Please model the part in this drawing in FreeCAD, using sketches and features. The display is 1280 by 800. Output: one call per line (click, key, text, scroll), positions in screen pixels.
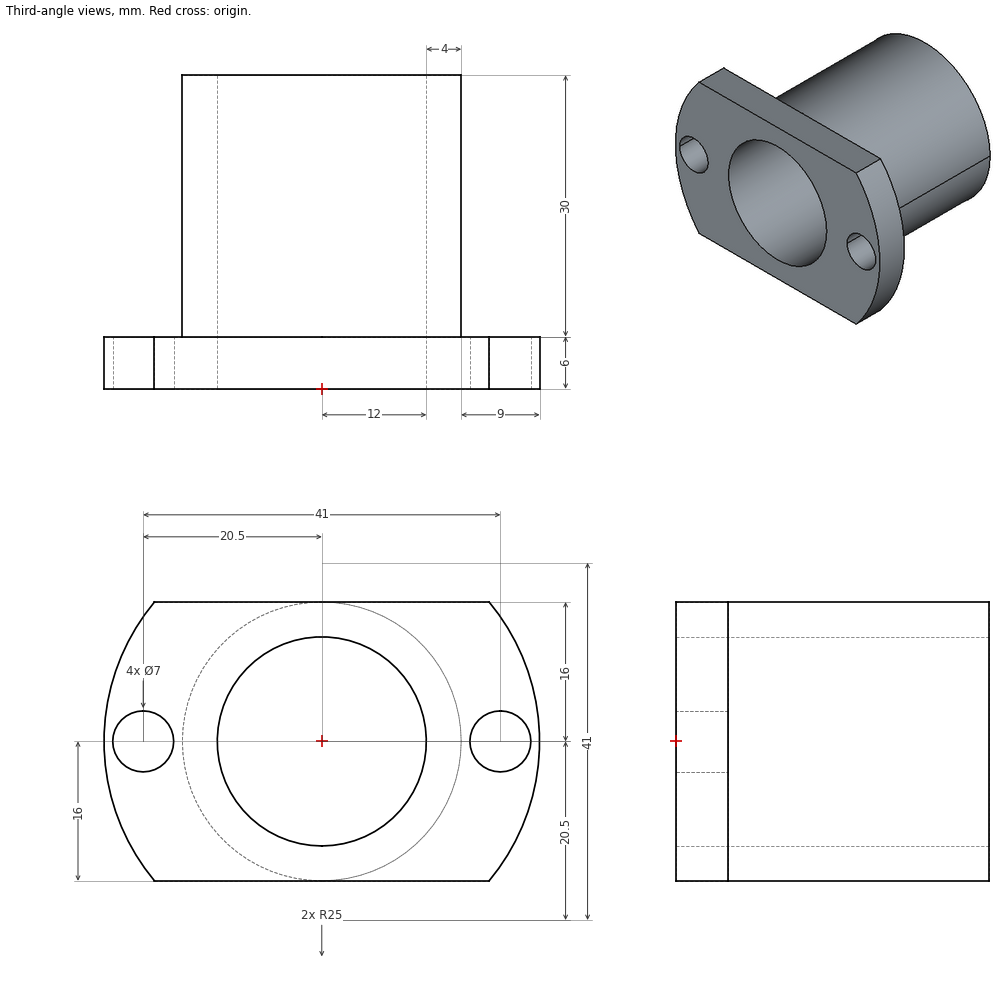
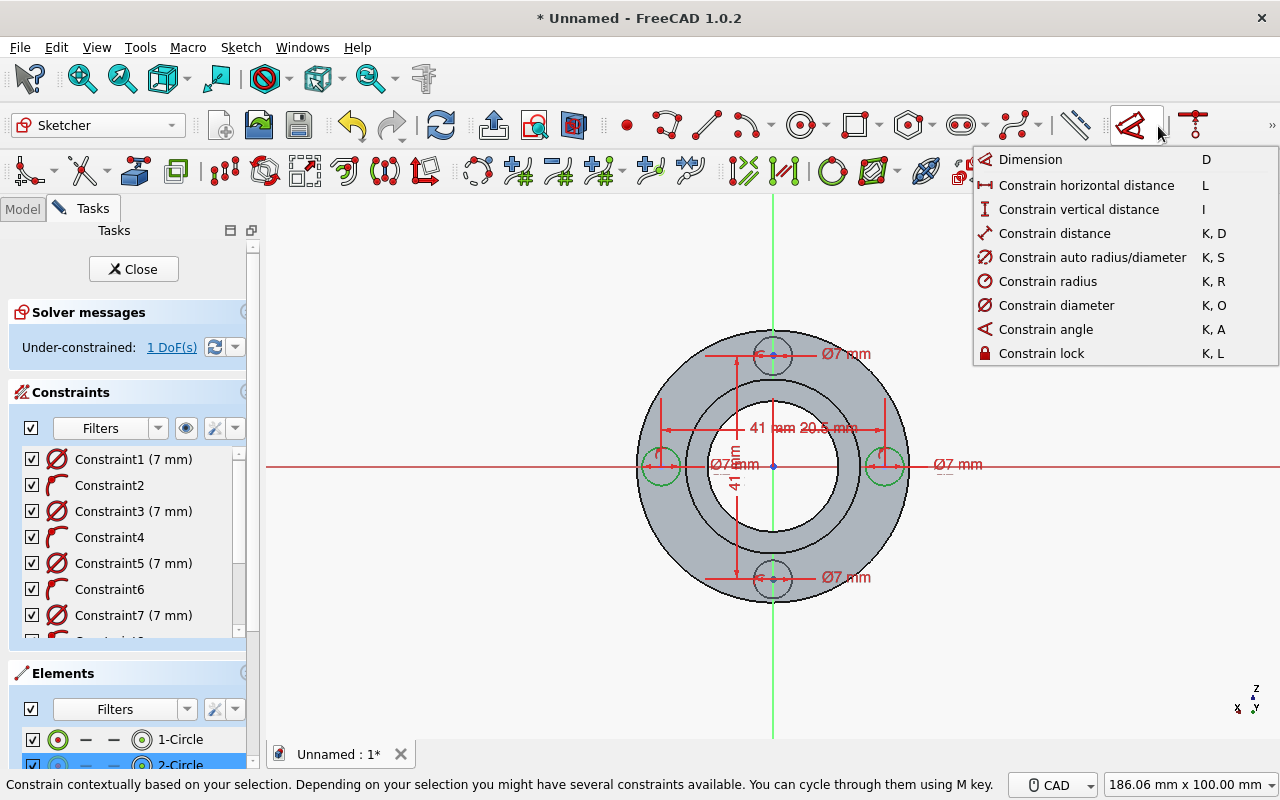
click(1126, 209)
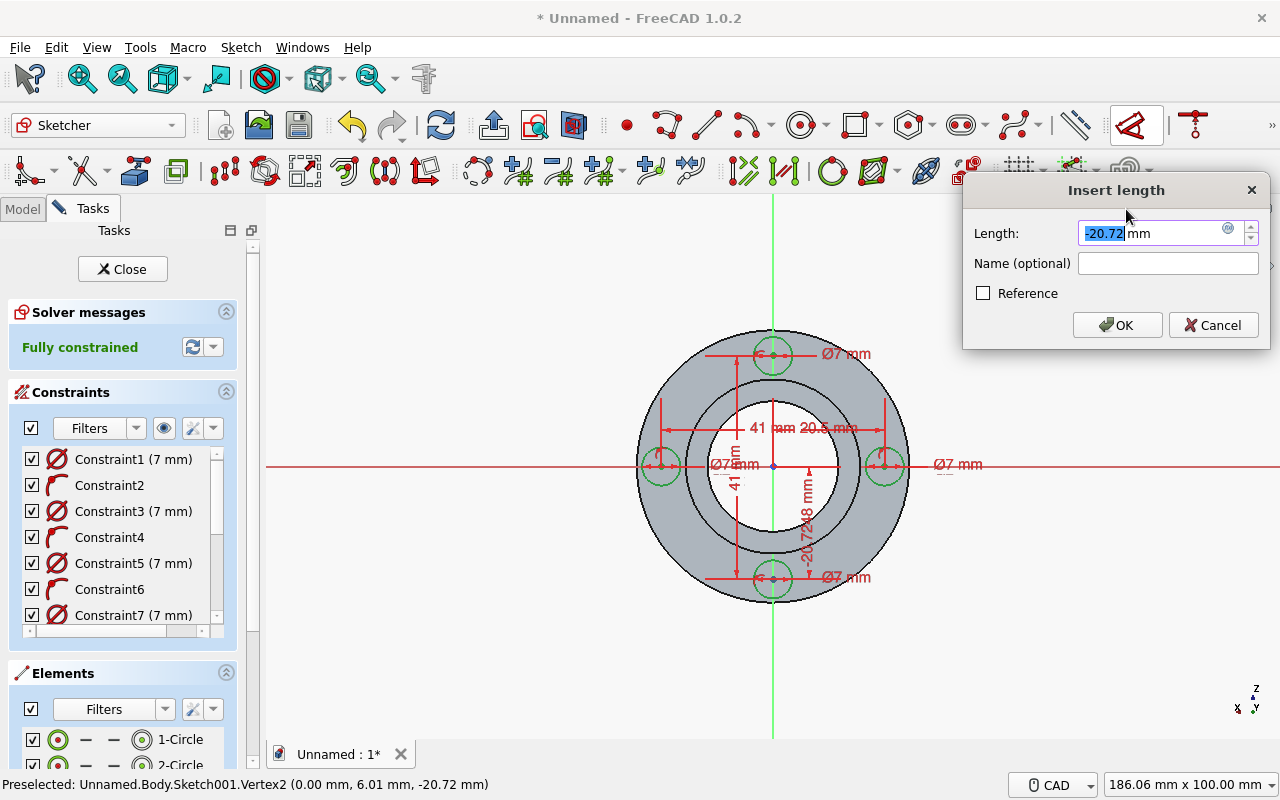
text(-20.5)
key(Return)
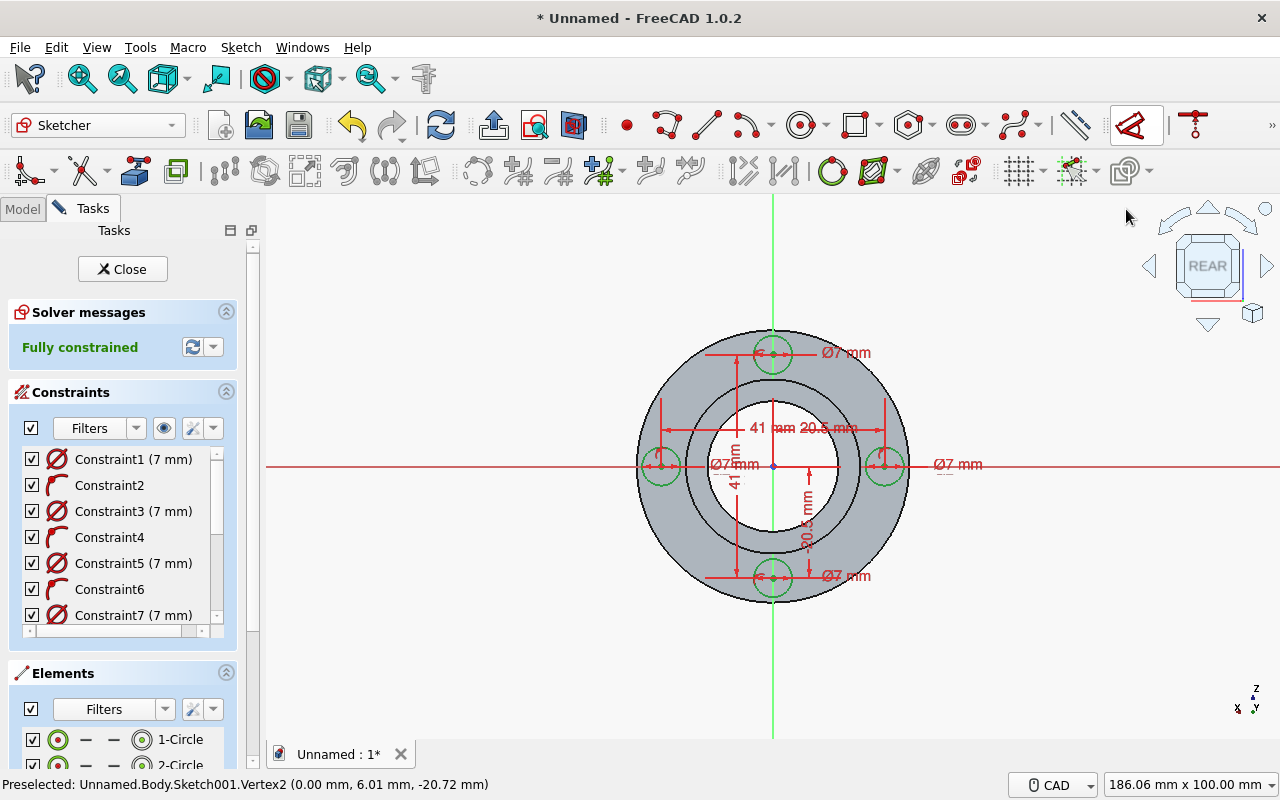
click(123, 269)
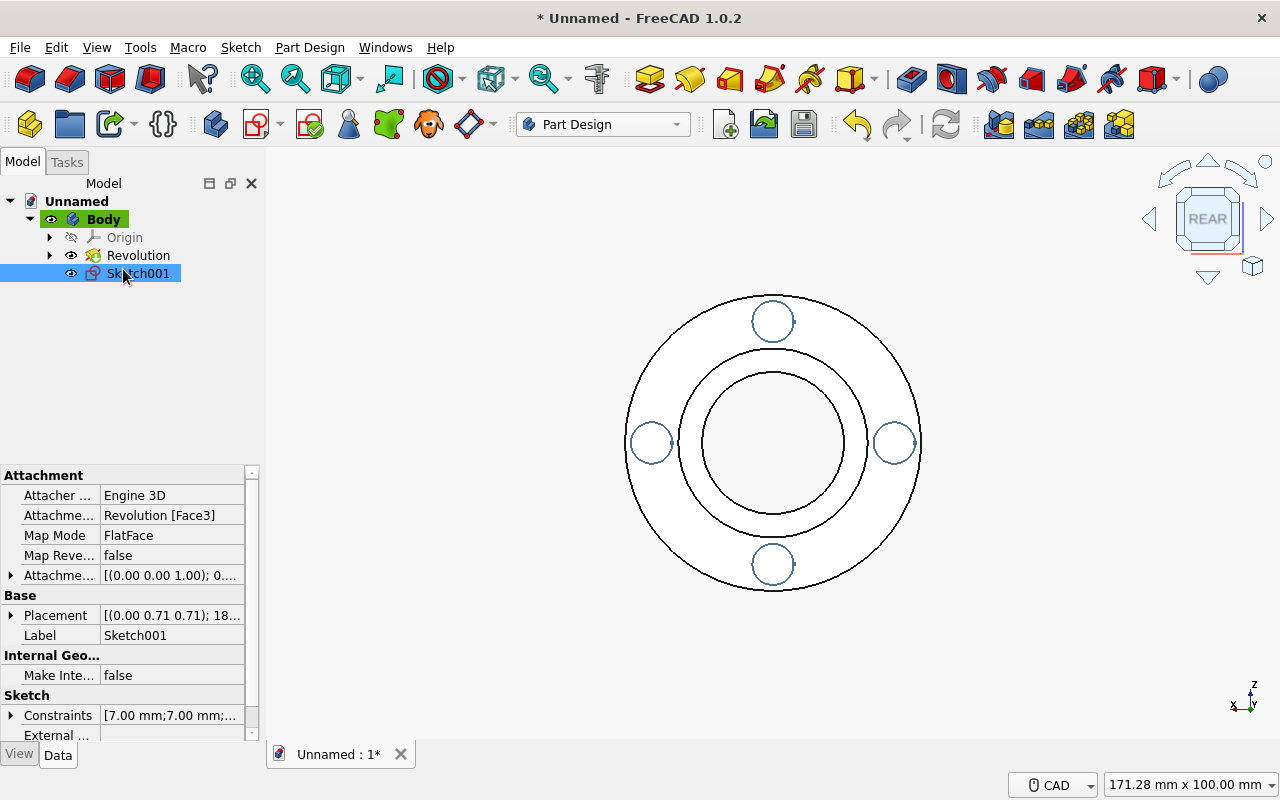
click(912, 80)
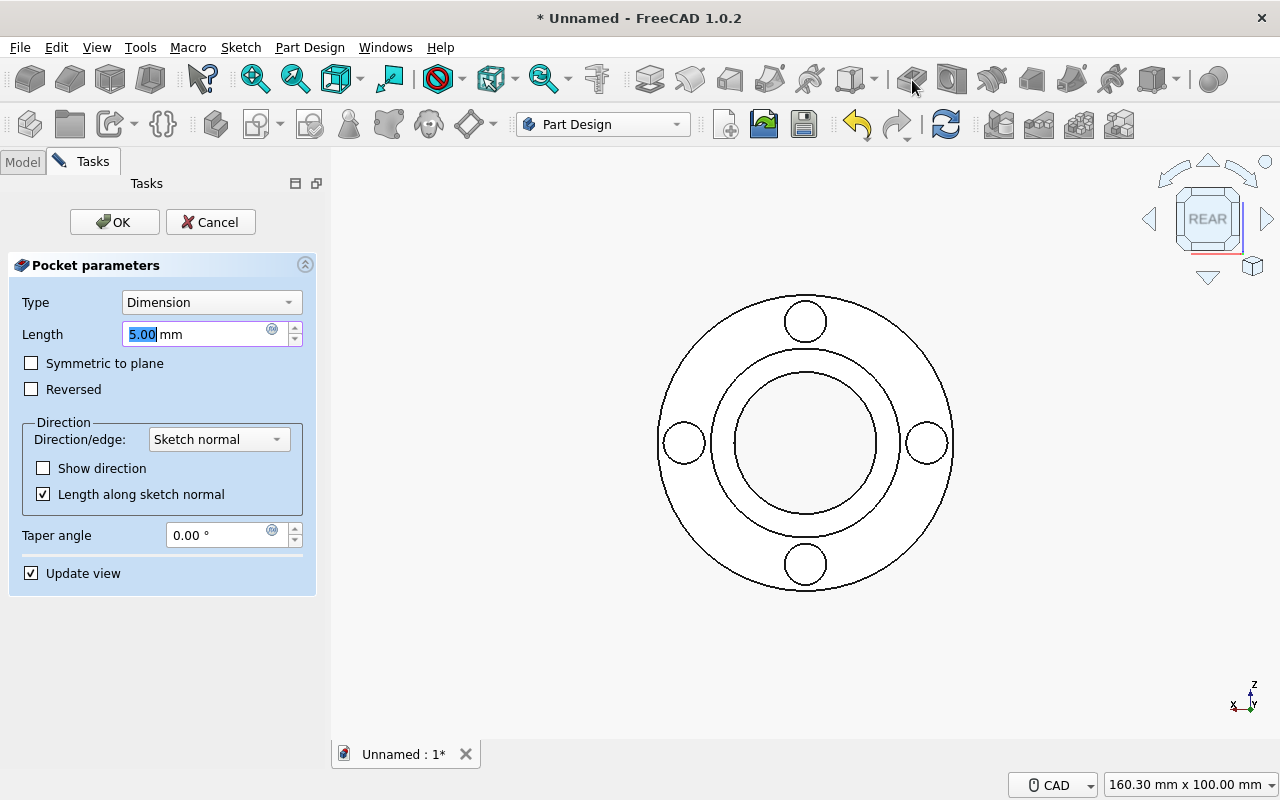
click(212, 302)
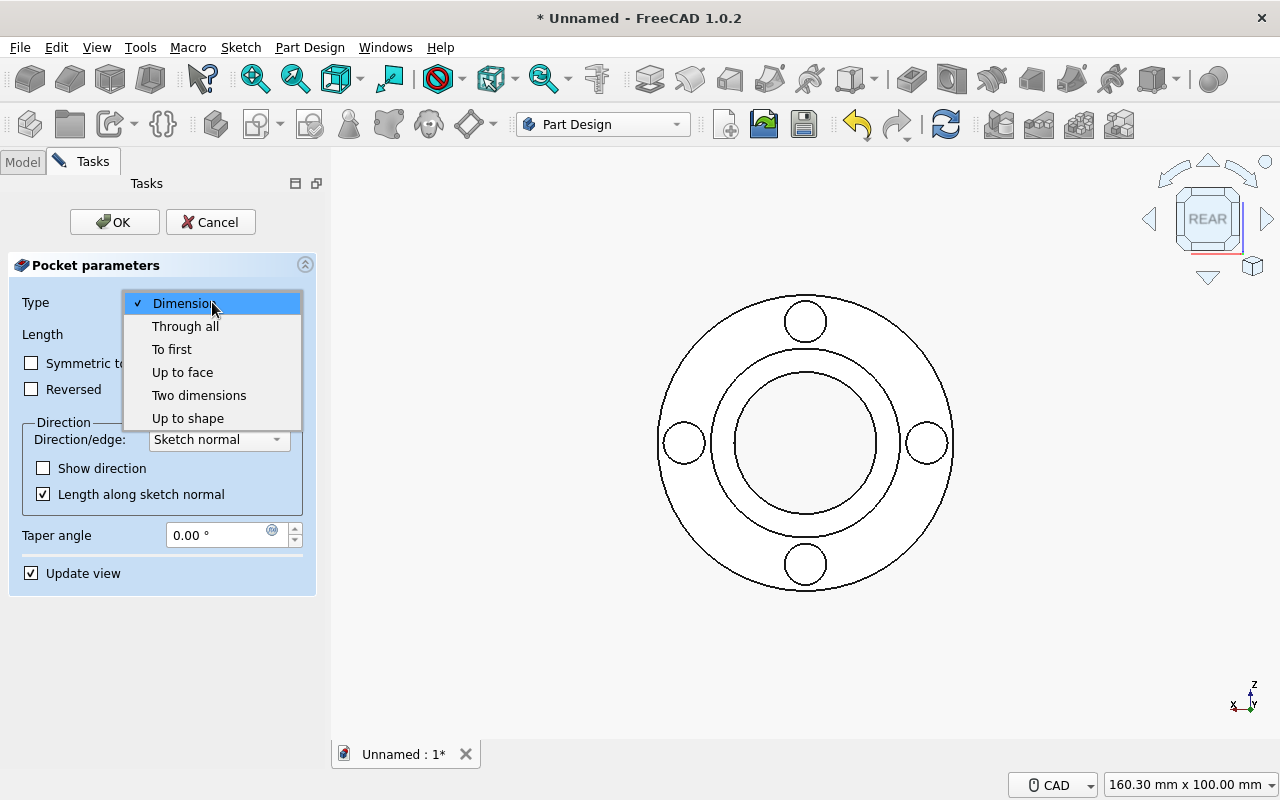
click(212, 326)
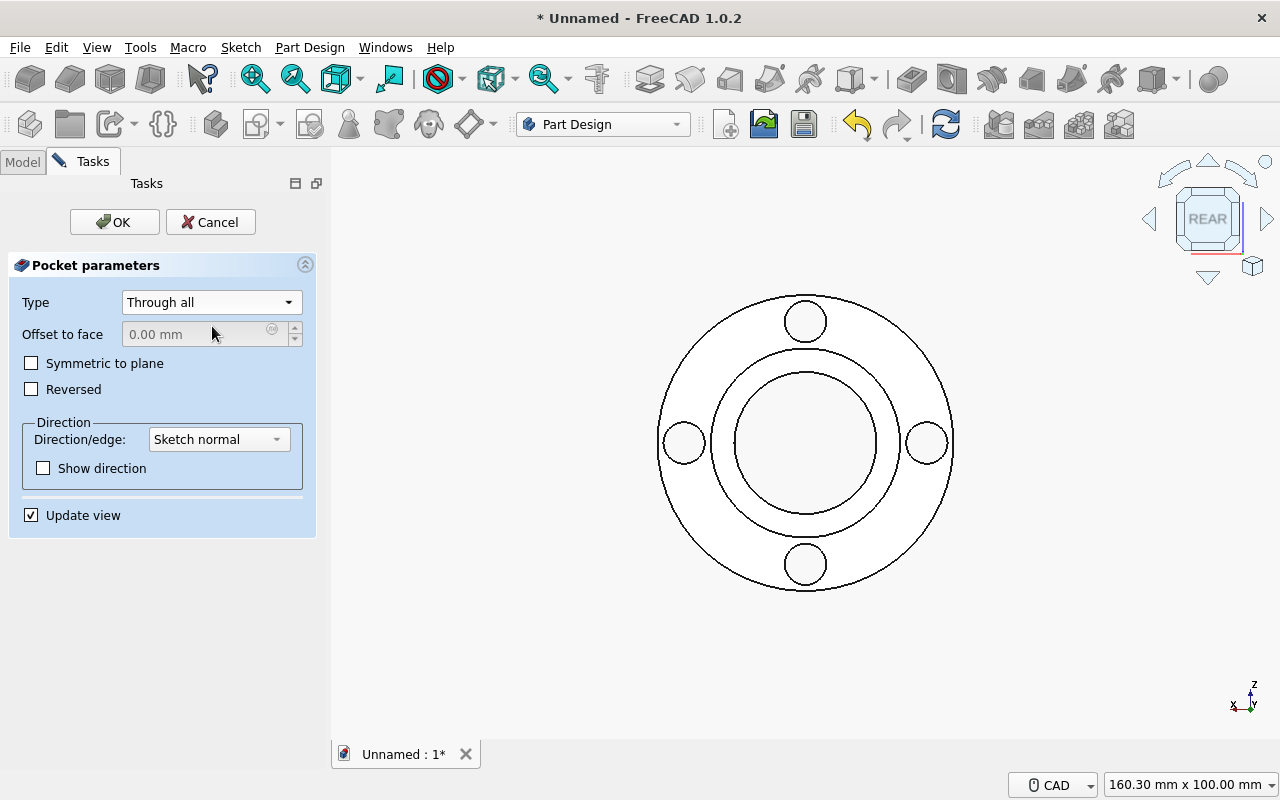
click(115, 222)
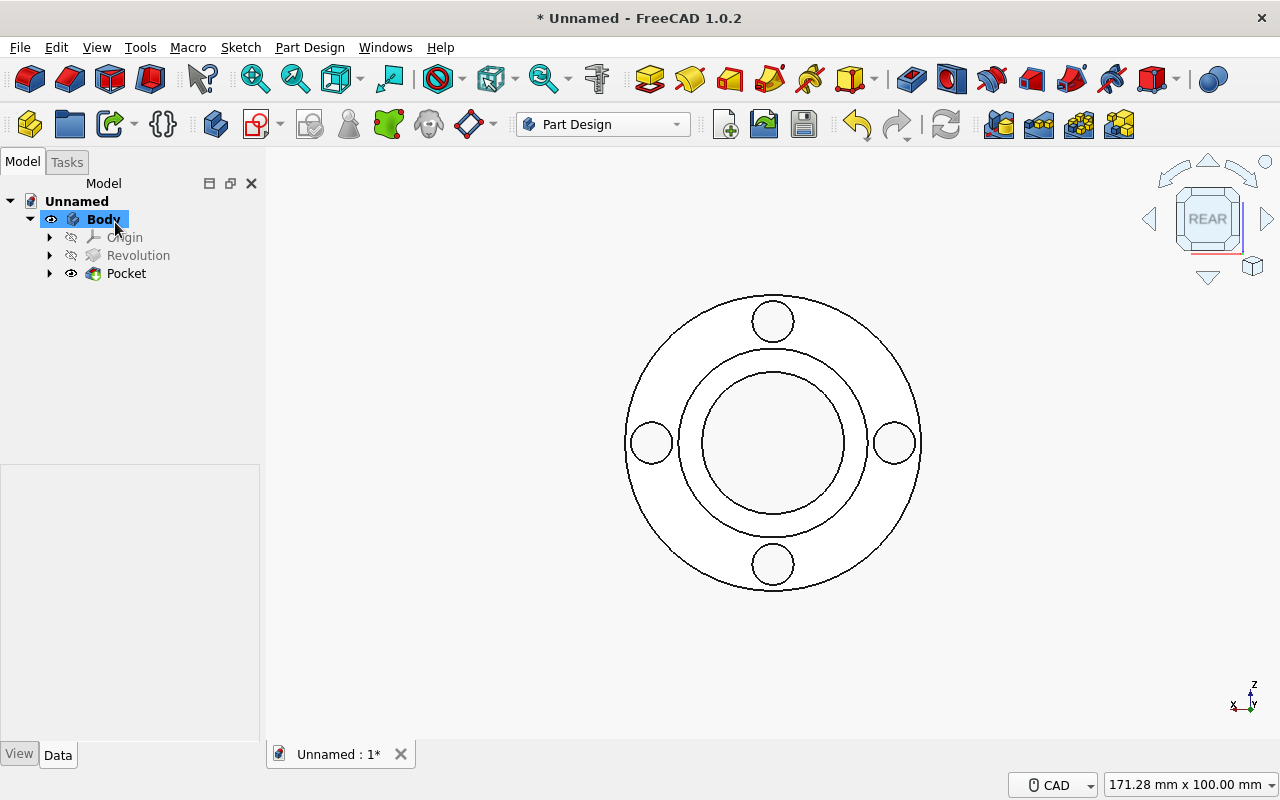
click(688, 527)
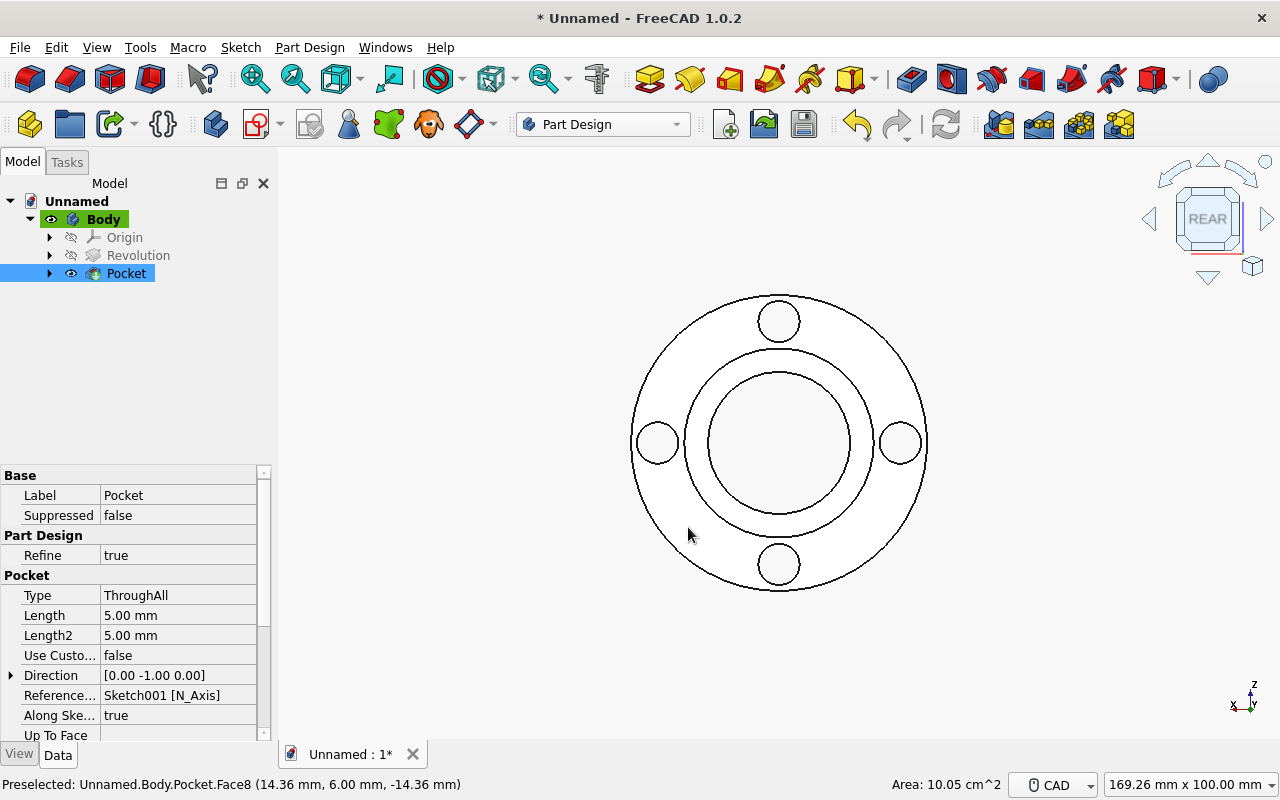
click(256, 124)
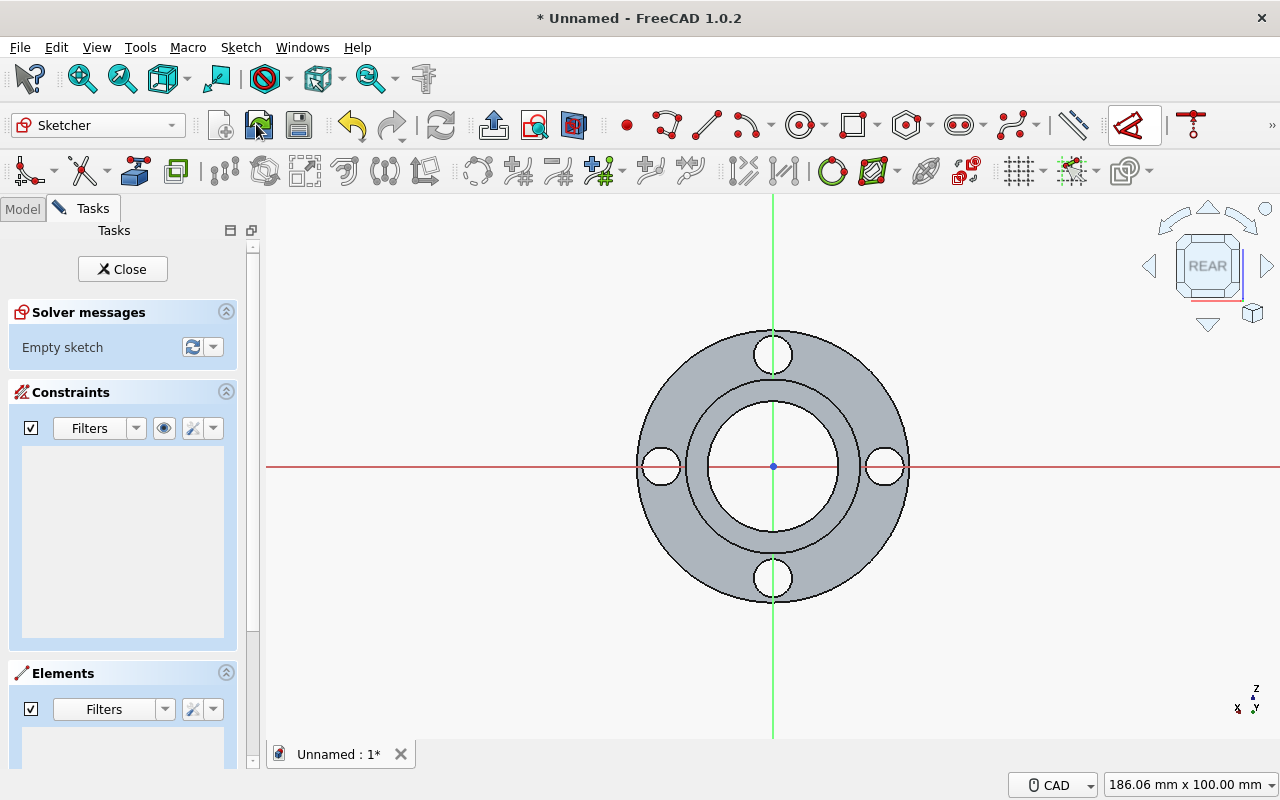
click(574, 126)